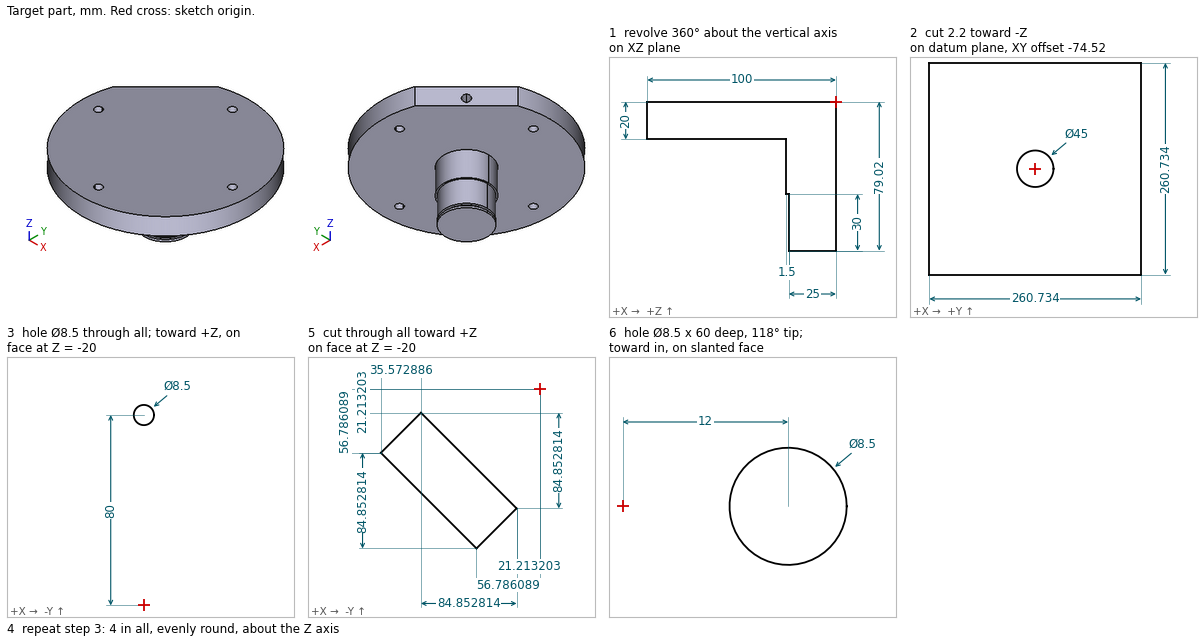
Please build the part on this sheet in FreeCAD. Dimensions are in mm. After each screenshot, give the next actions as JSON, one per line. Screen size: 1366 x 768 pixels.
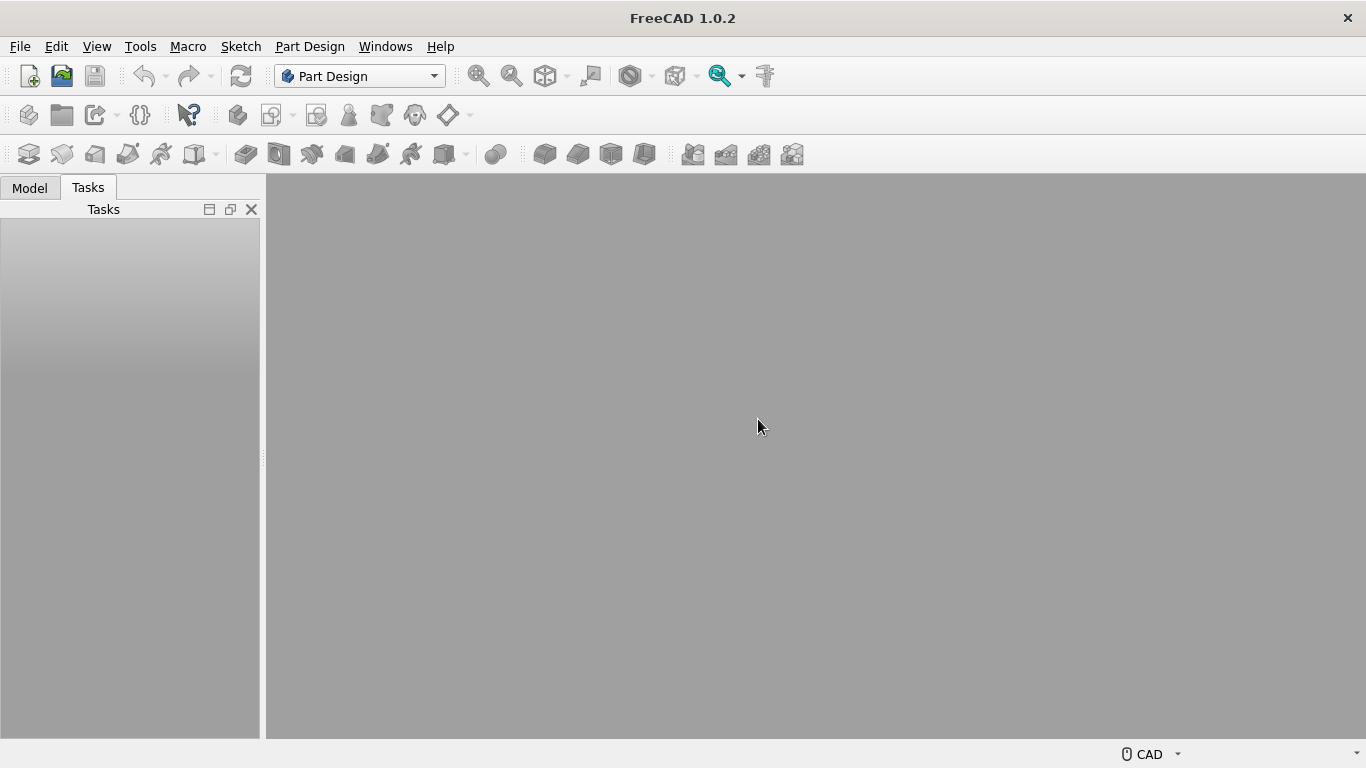
{"action": "left_click", "coordinate": [29, 76]}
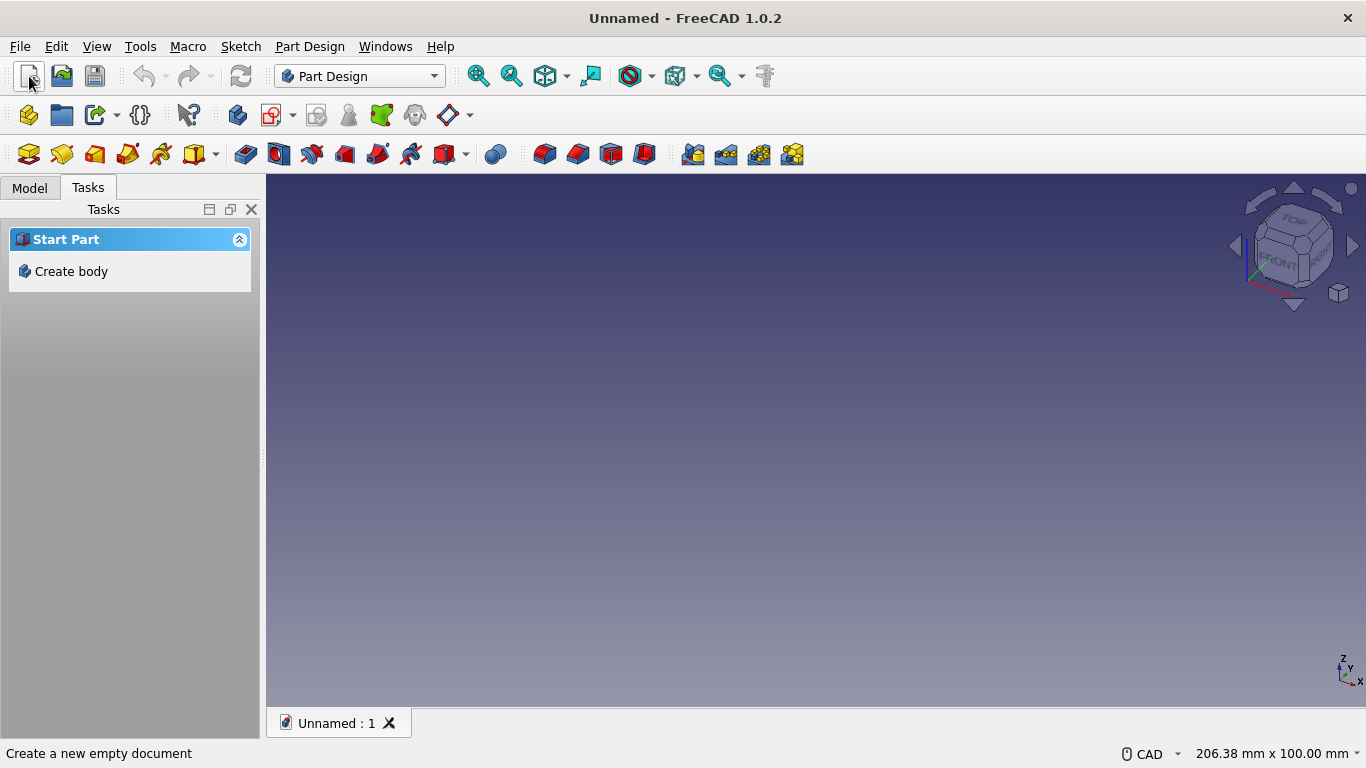
{"action": "left_click", "coordinate": [270, 116]}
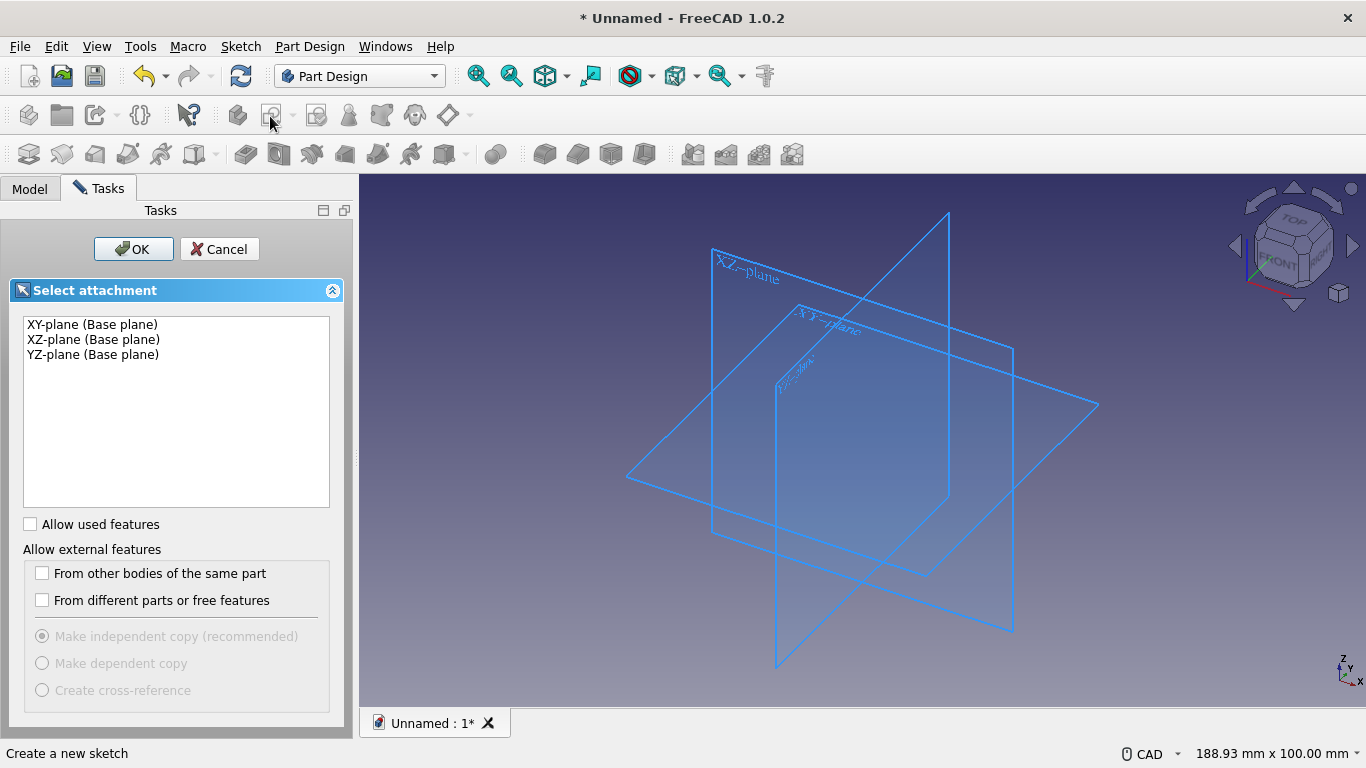
{"action": "left_click", "coordinate": [84, 340]}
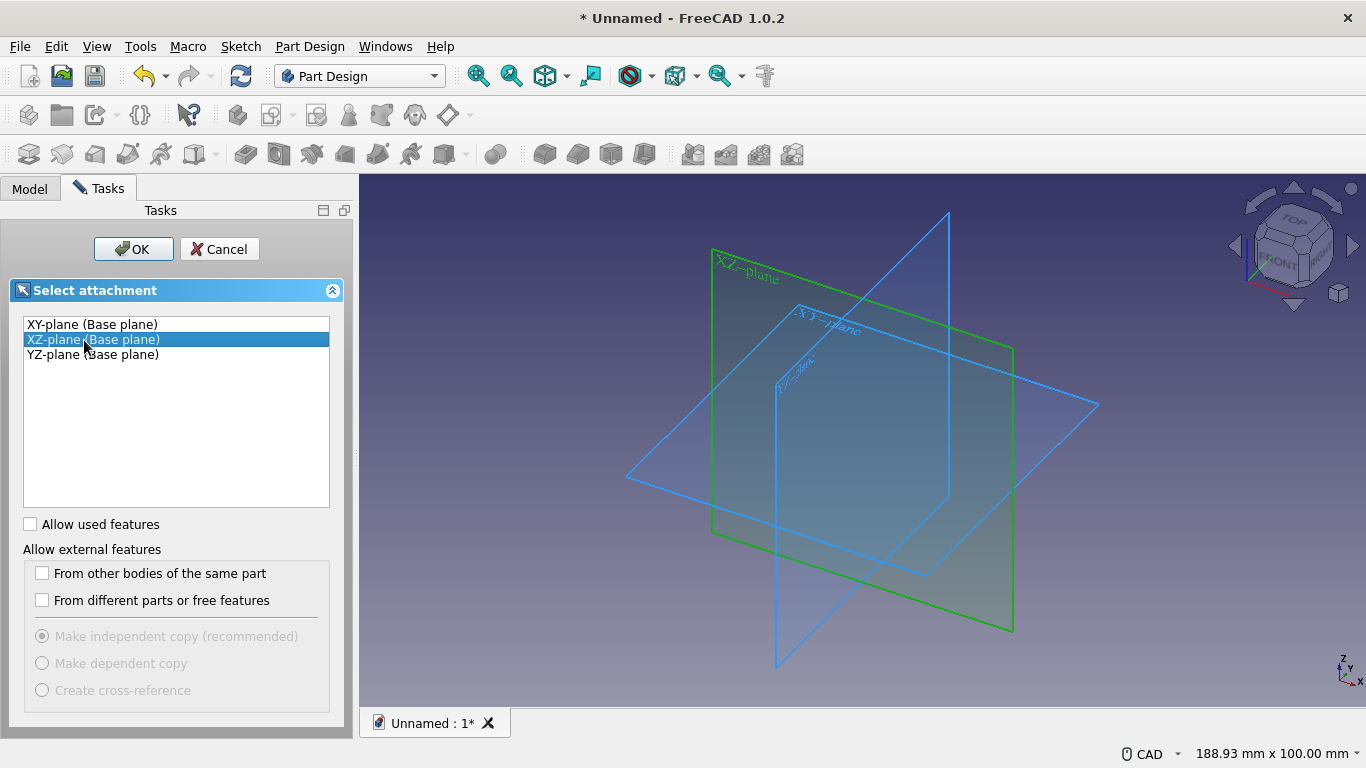
{"action": "left_click", "coordinate": [134, 249]}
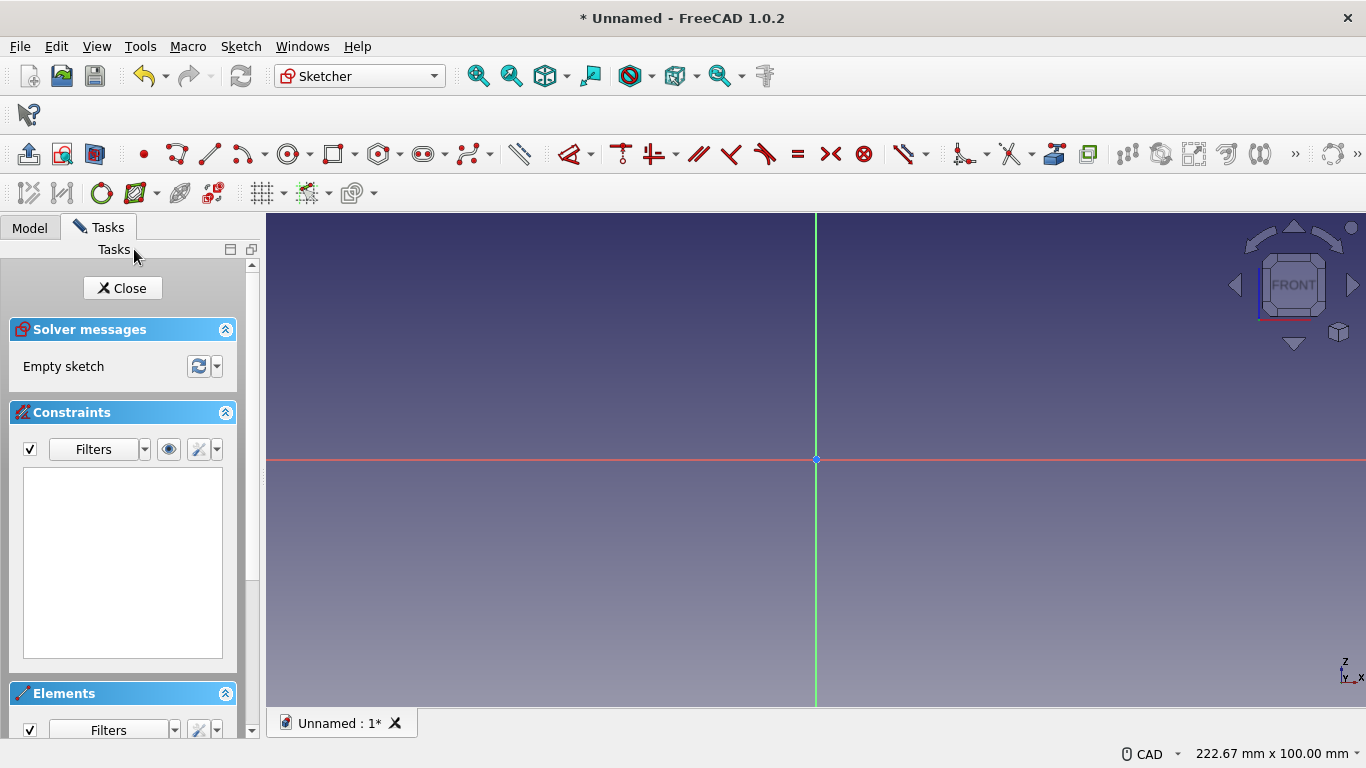
{"action": "scroll", "coordinate": [1110, 241], "scroll_direction": "down", "scroll_amount": 2}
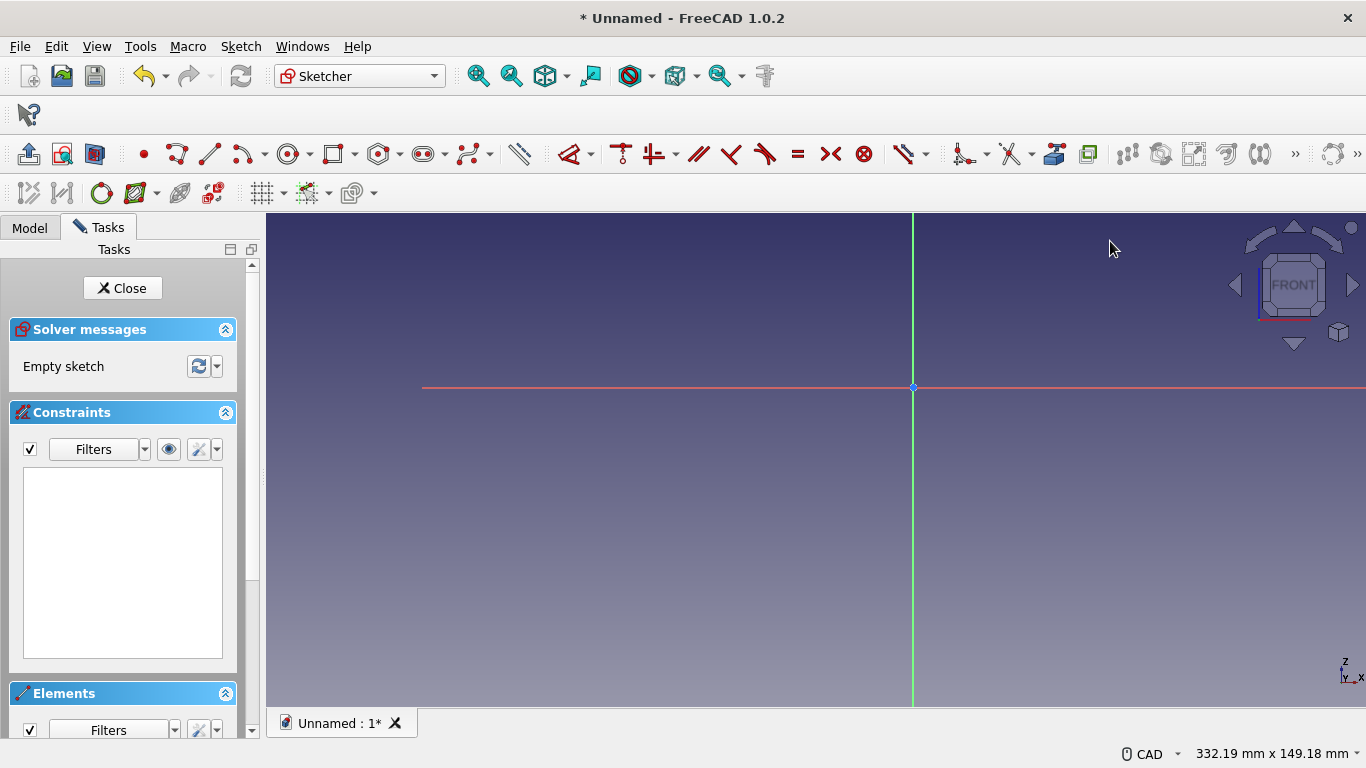
{"action": "left_click", "coordinate": [177, 154]}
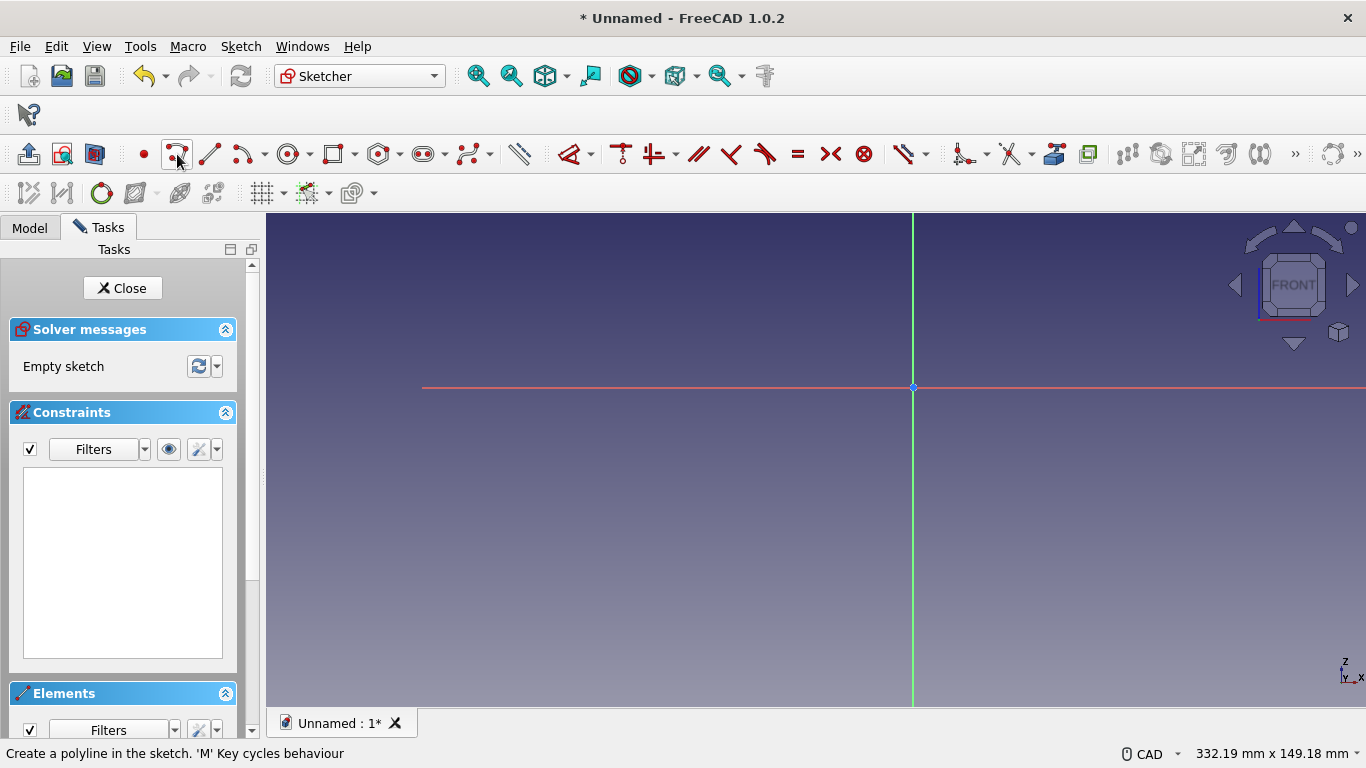
{"action": "left_click", "coordinate": [913, 388]}
{"action": "left_click", "coordinate": [904, 649]}
{"action": "left_click", "coordinate": [830, 649]}
{"action": "left_click", "coordinate": [830, 550]}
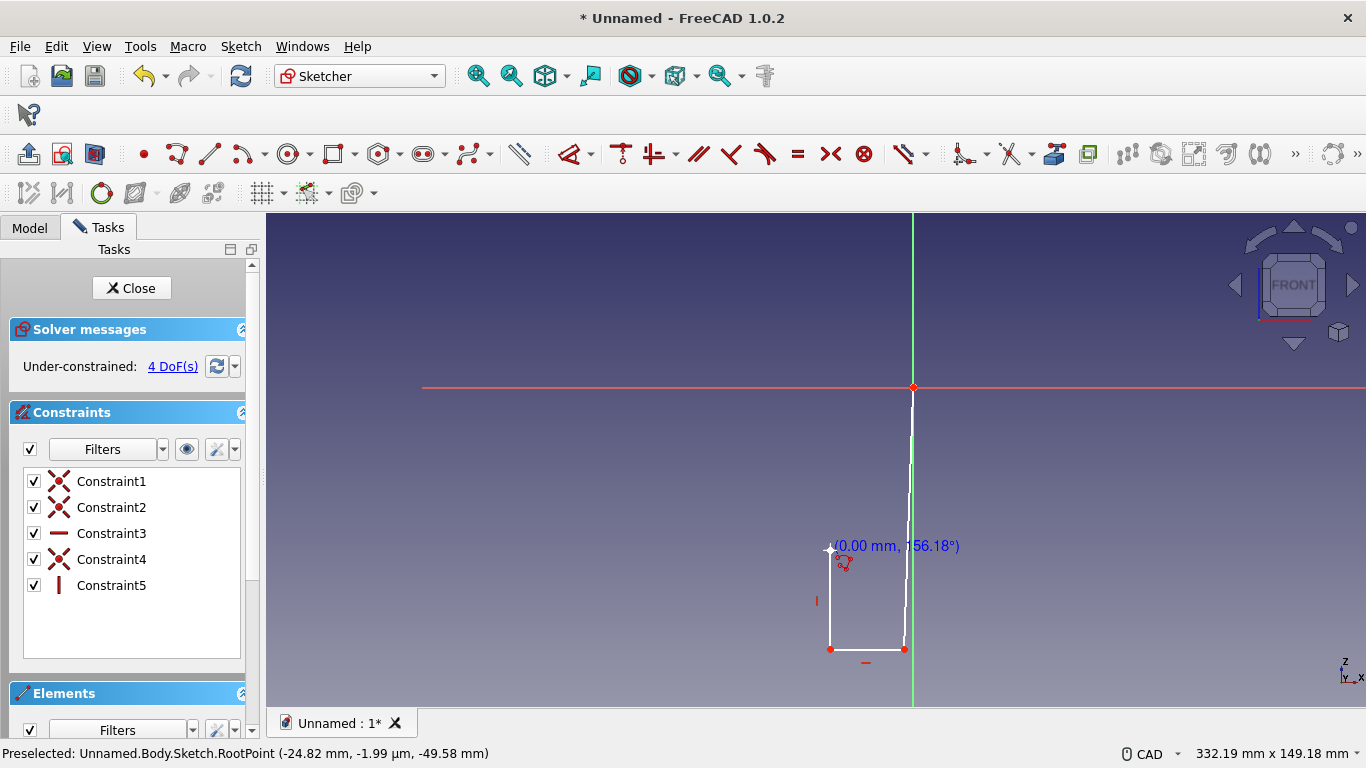
{"action": "scroll", "coordinate": [825, 550], "scroll_direction": "up", "scroll_amount": 6}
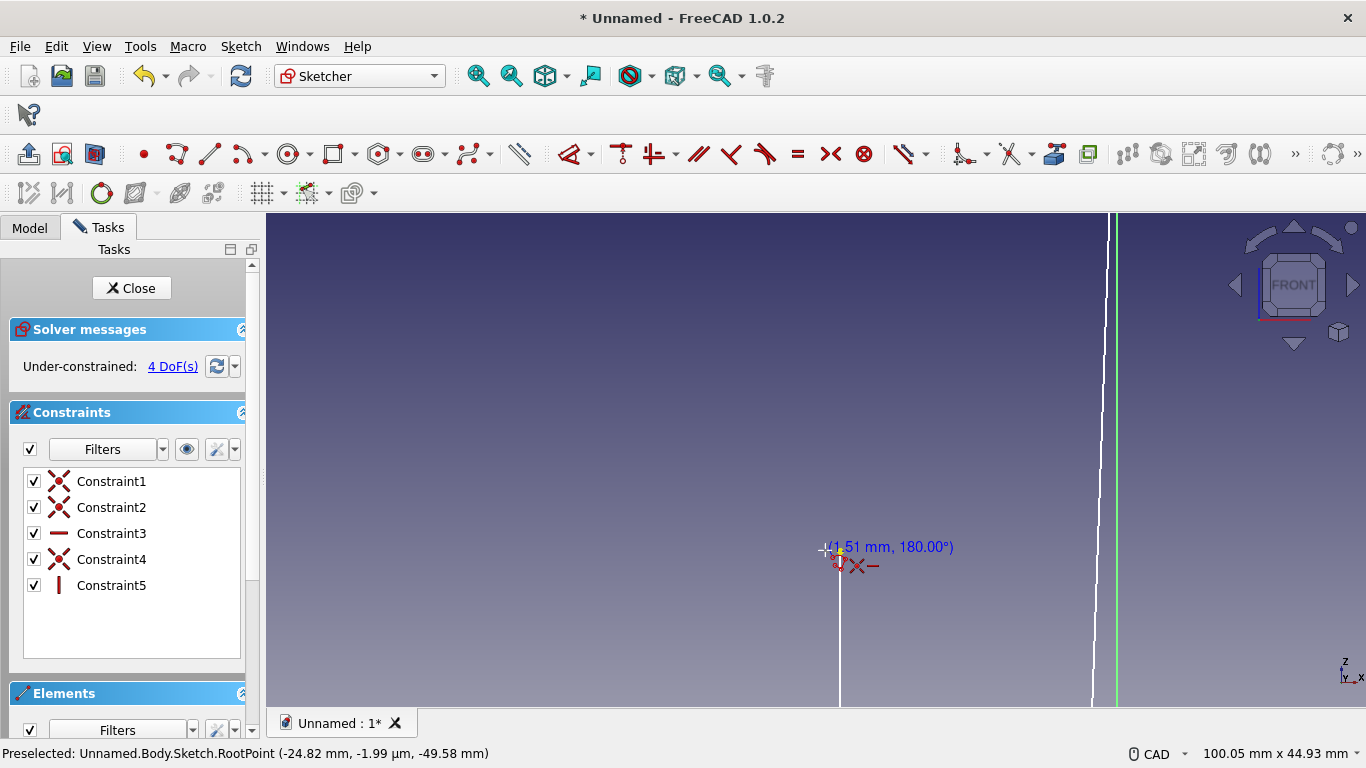
{"action": "left_click", "coordinate": [825, 548]}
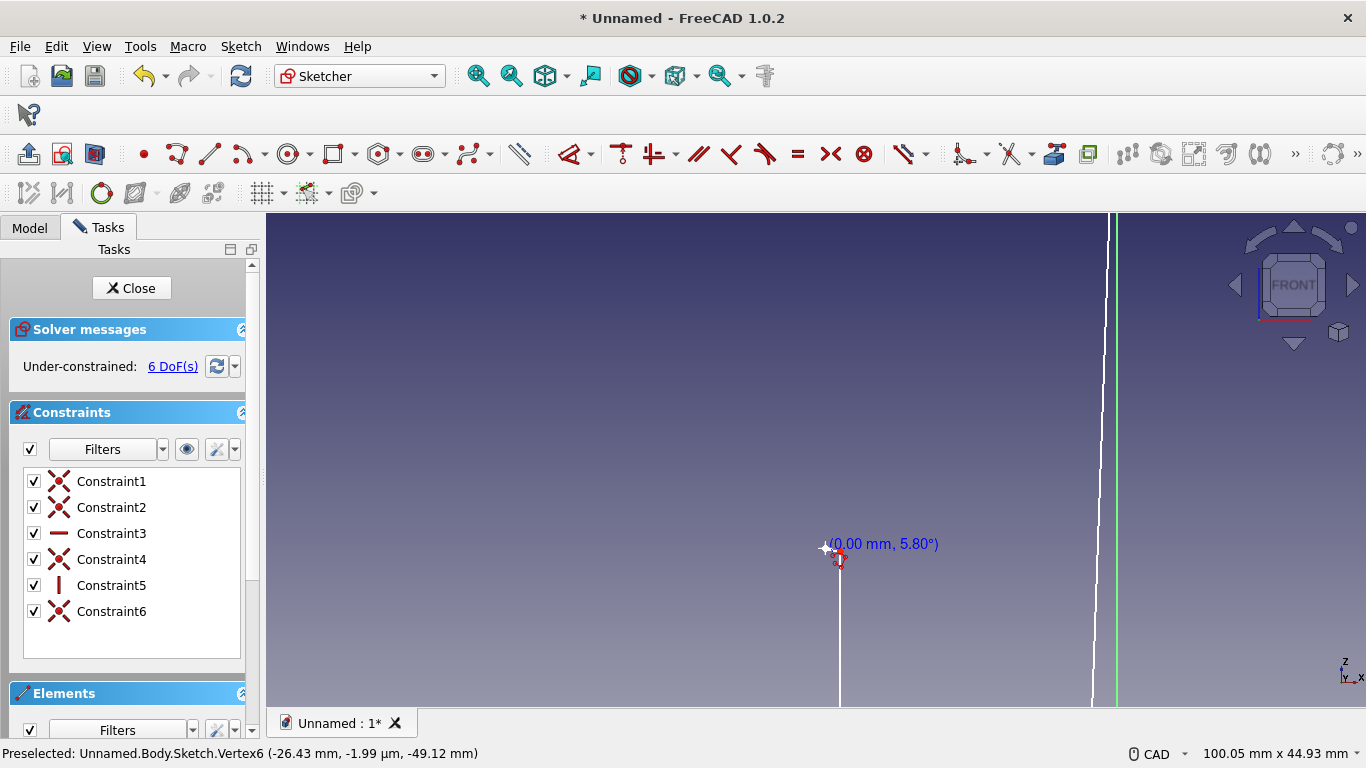
{"action": "scroll", "coordinate": [853, 469], "scroll_direction": "down", "scroll_amount": 5}